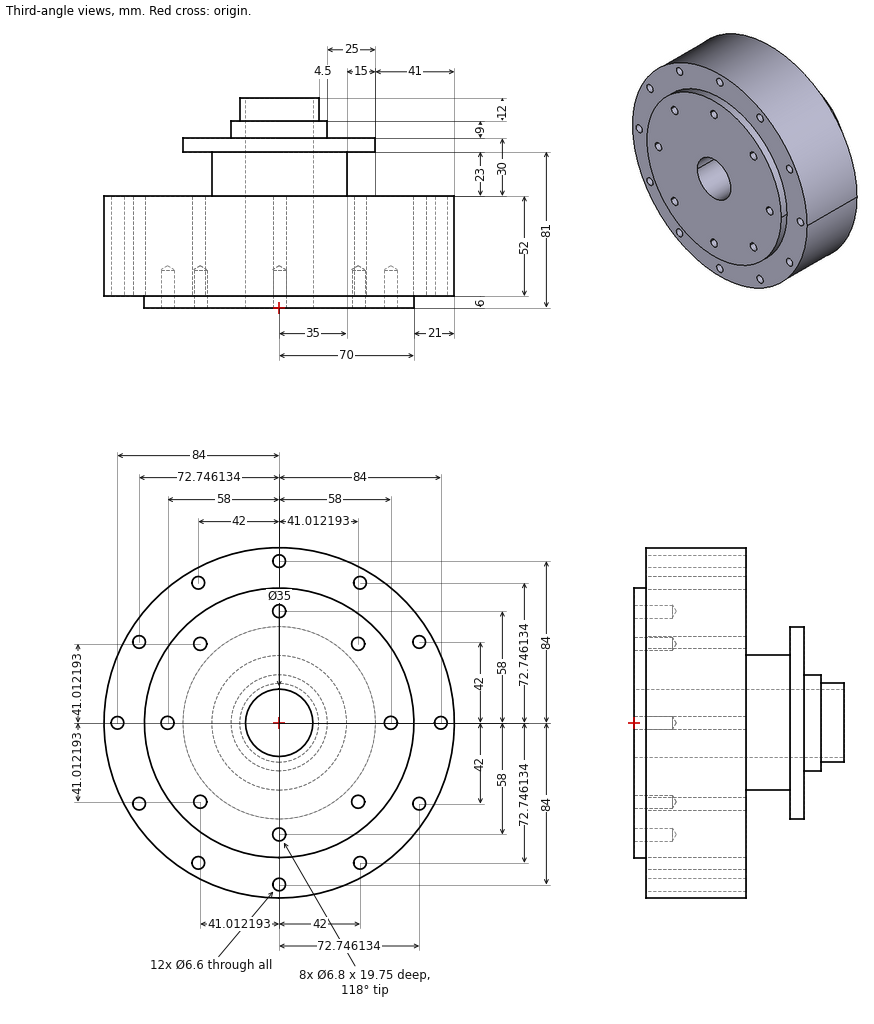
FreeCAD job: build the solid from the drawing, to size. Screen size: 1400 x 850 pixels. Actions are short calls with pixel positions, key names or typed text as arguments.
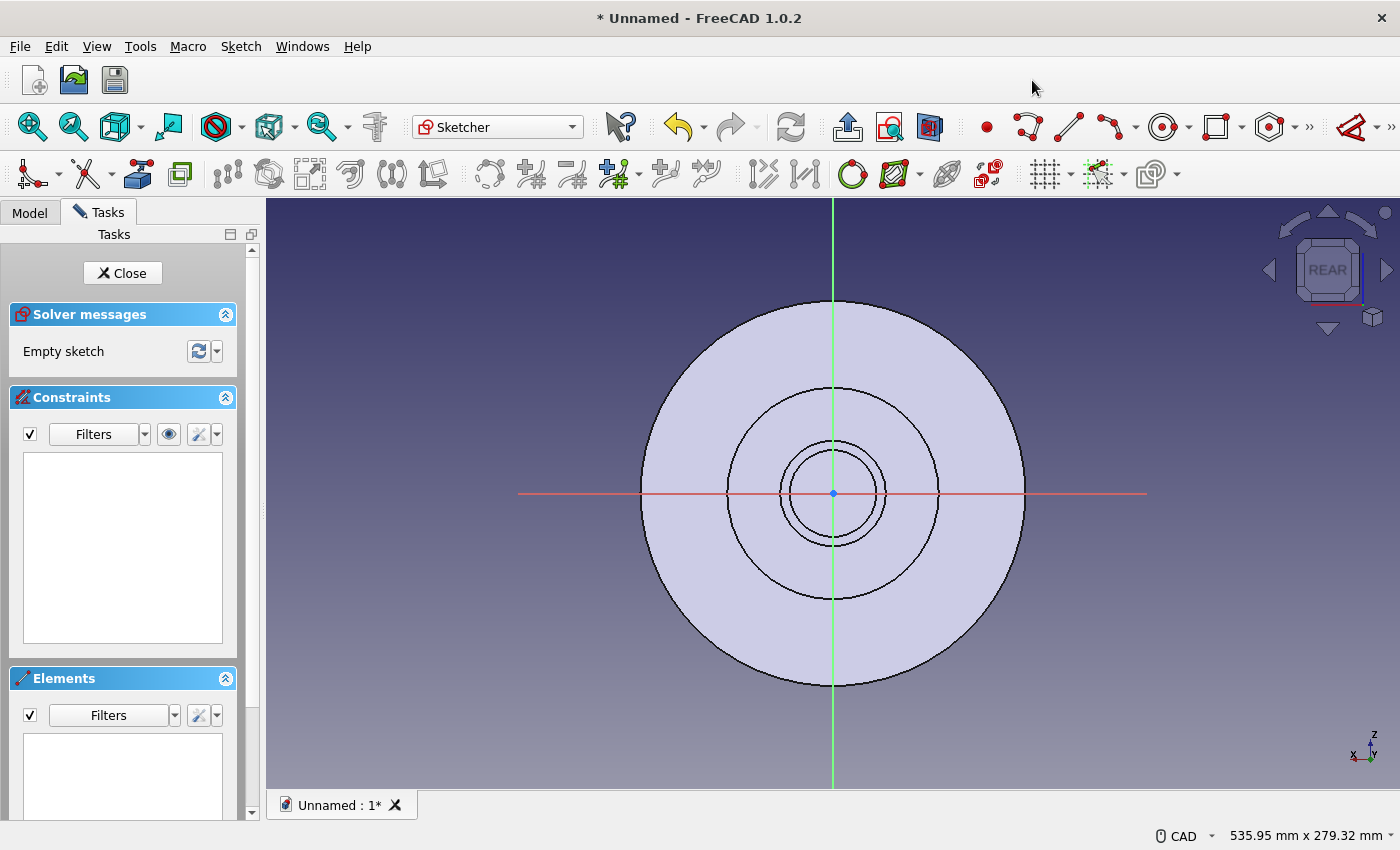
scroll(850, 493, up, 8)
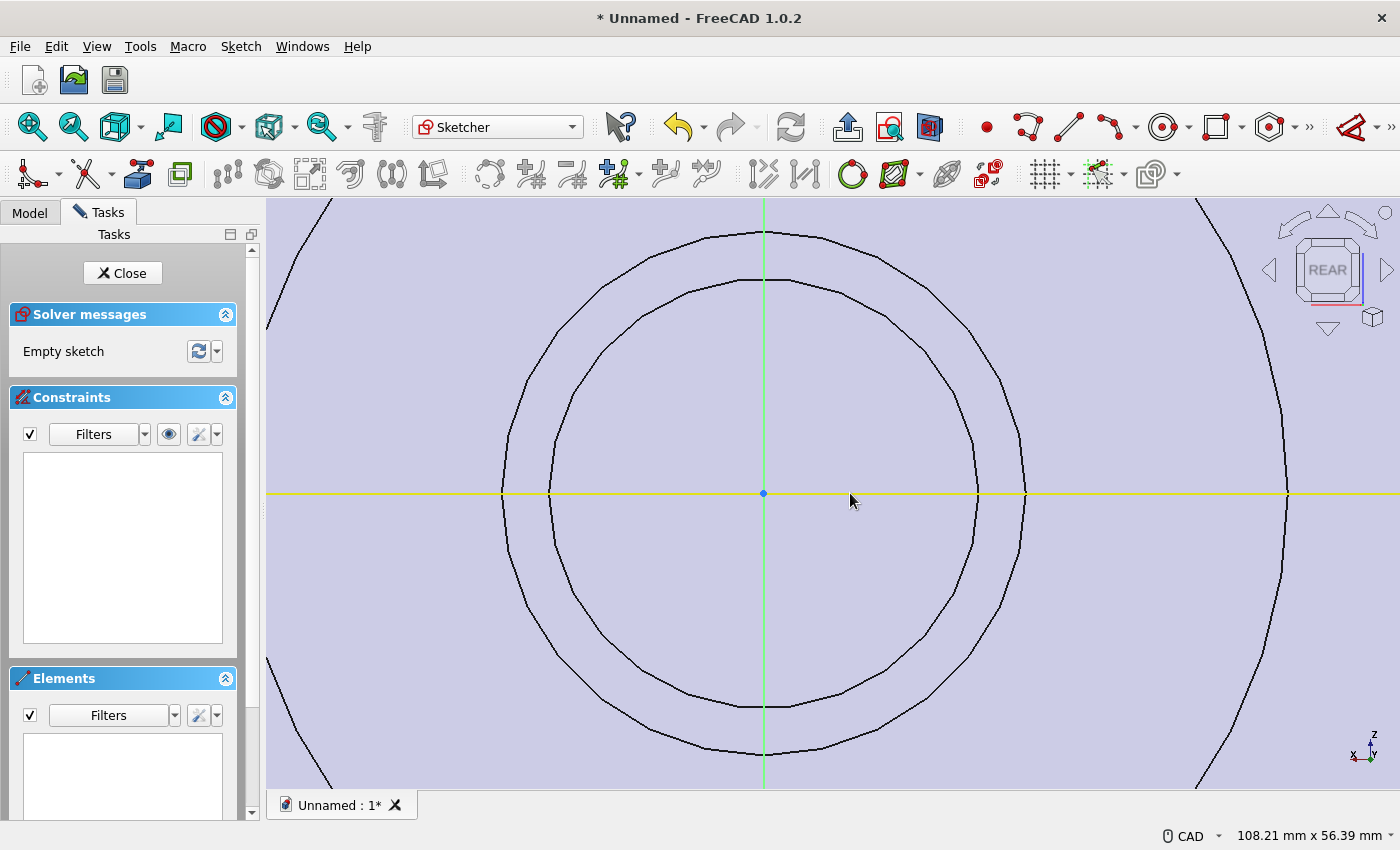
key(g)
key(c)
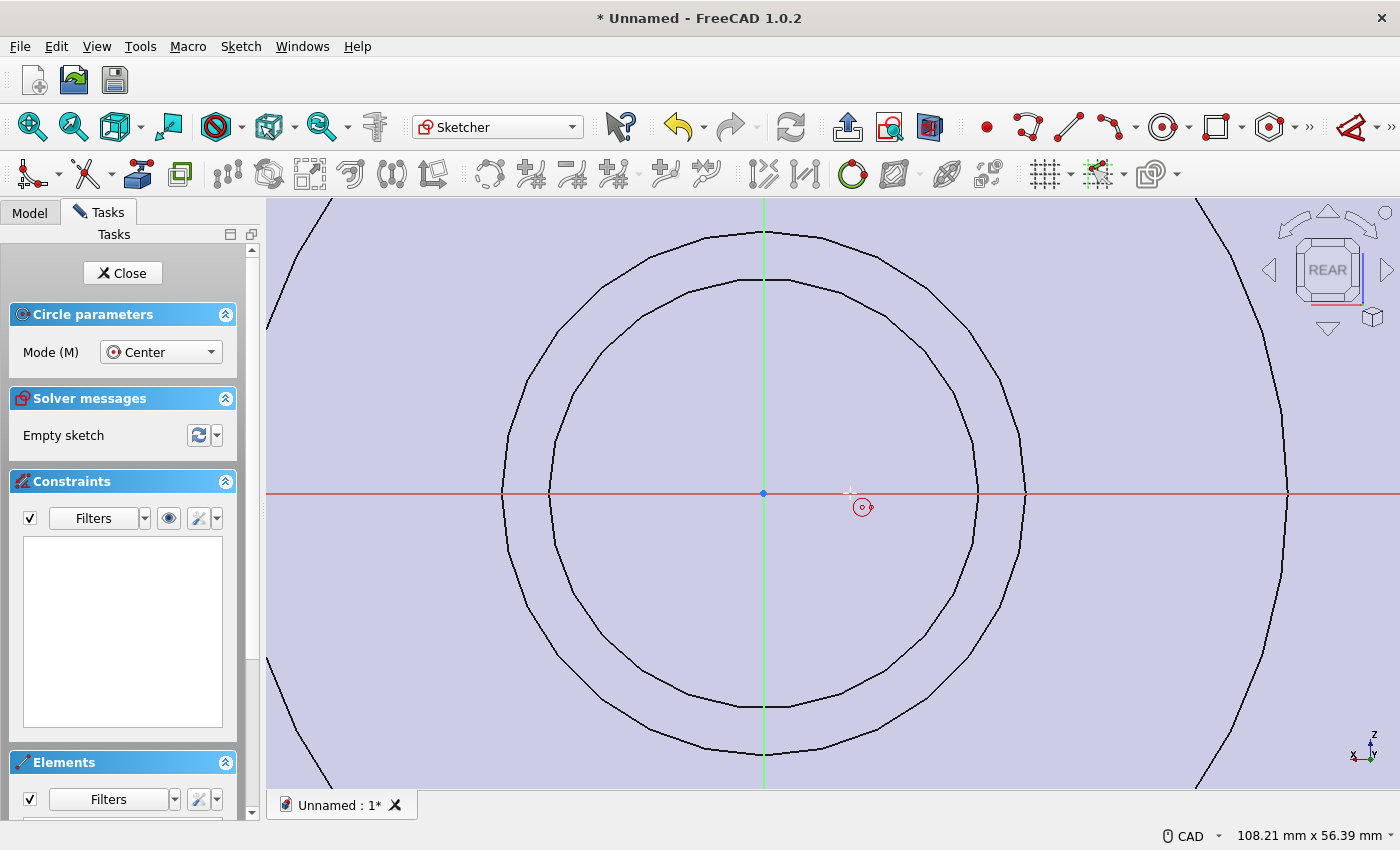
click(764, 493)
click(893, 364)
key(Escape)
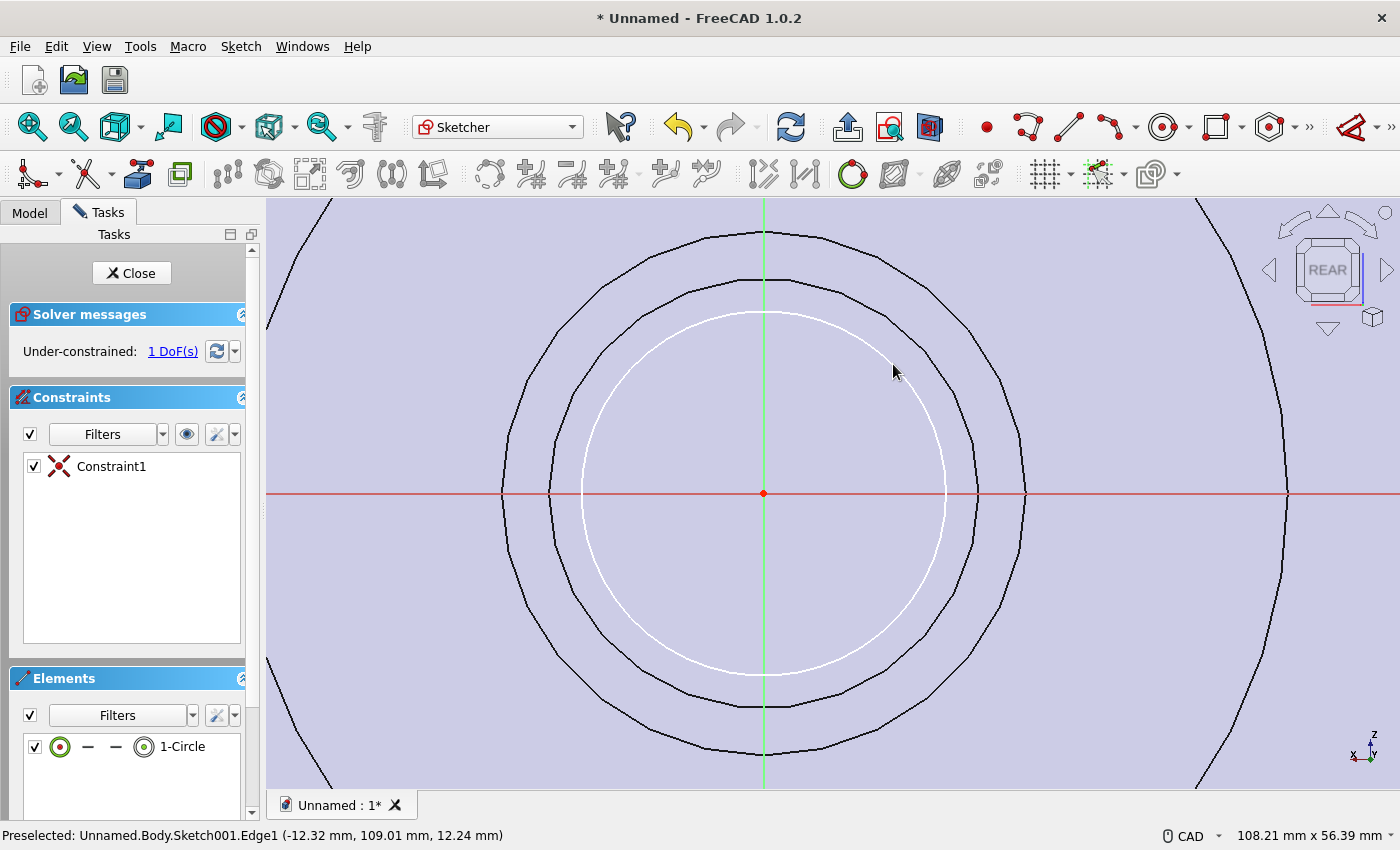
key(d)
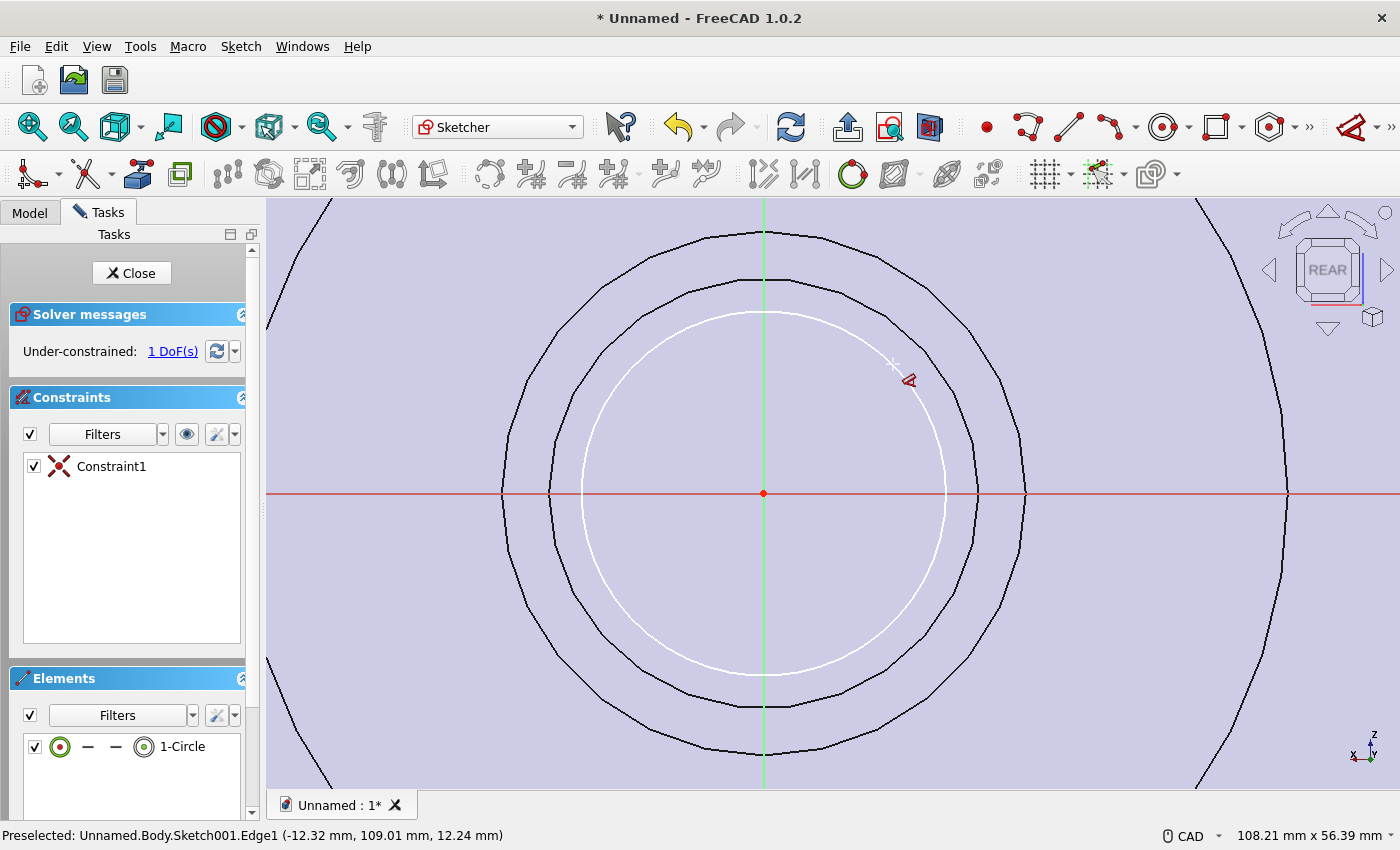
click(892, 364)
click(915, 341)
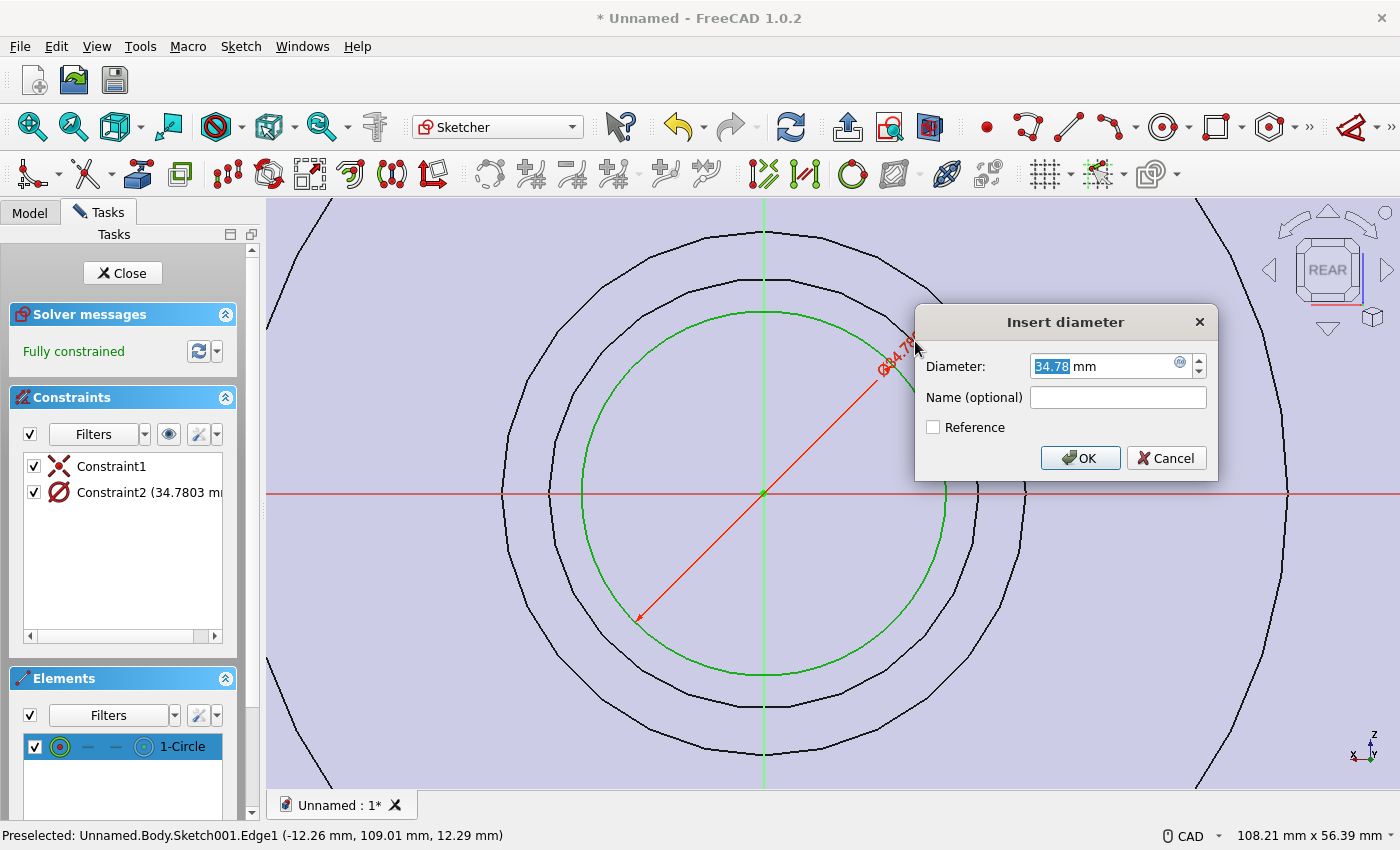
text(35)
key(Return)
key(Escape)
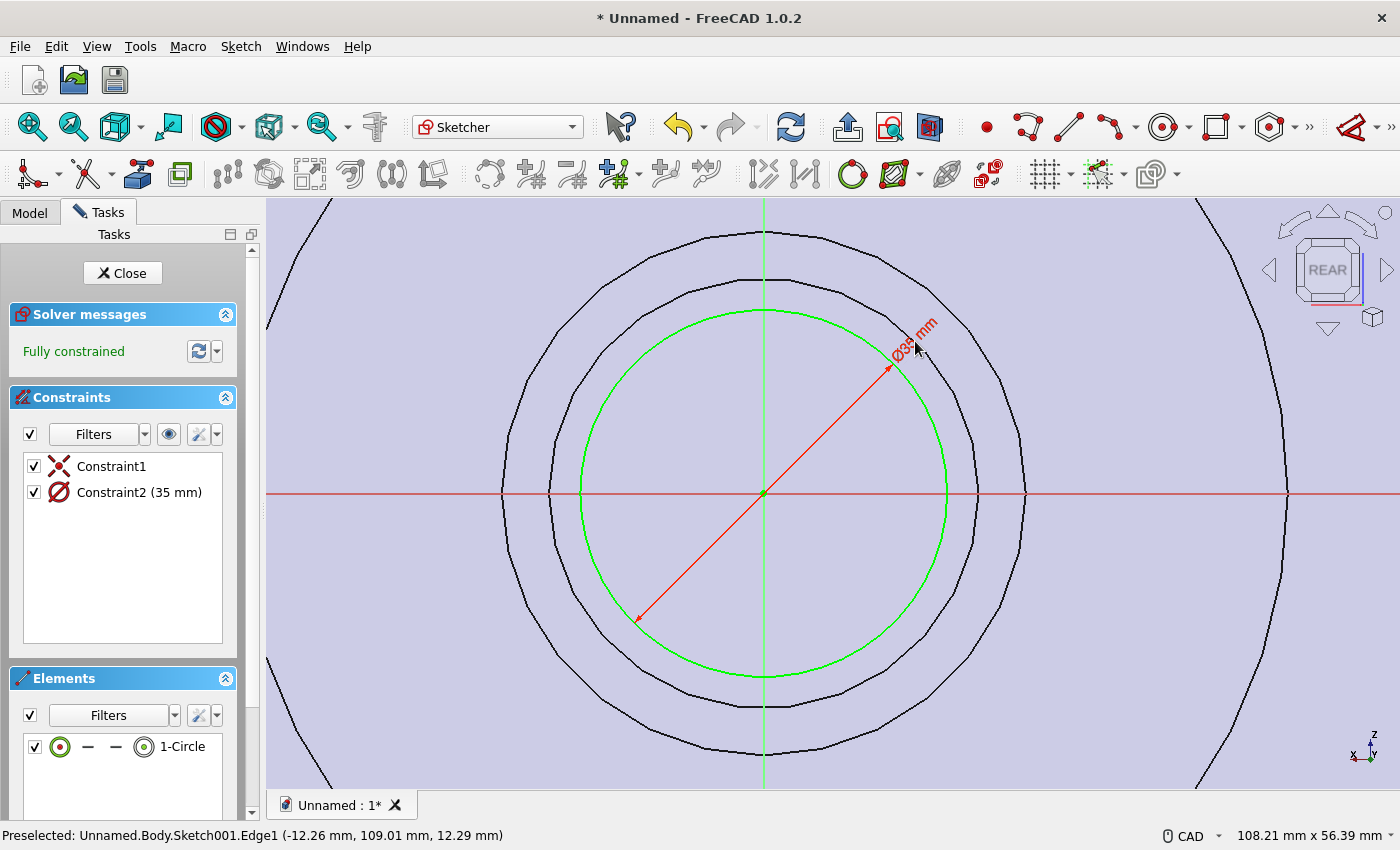
click(123, 273)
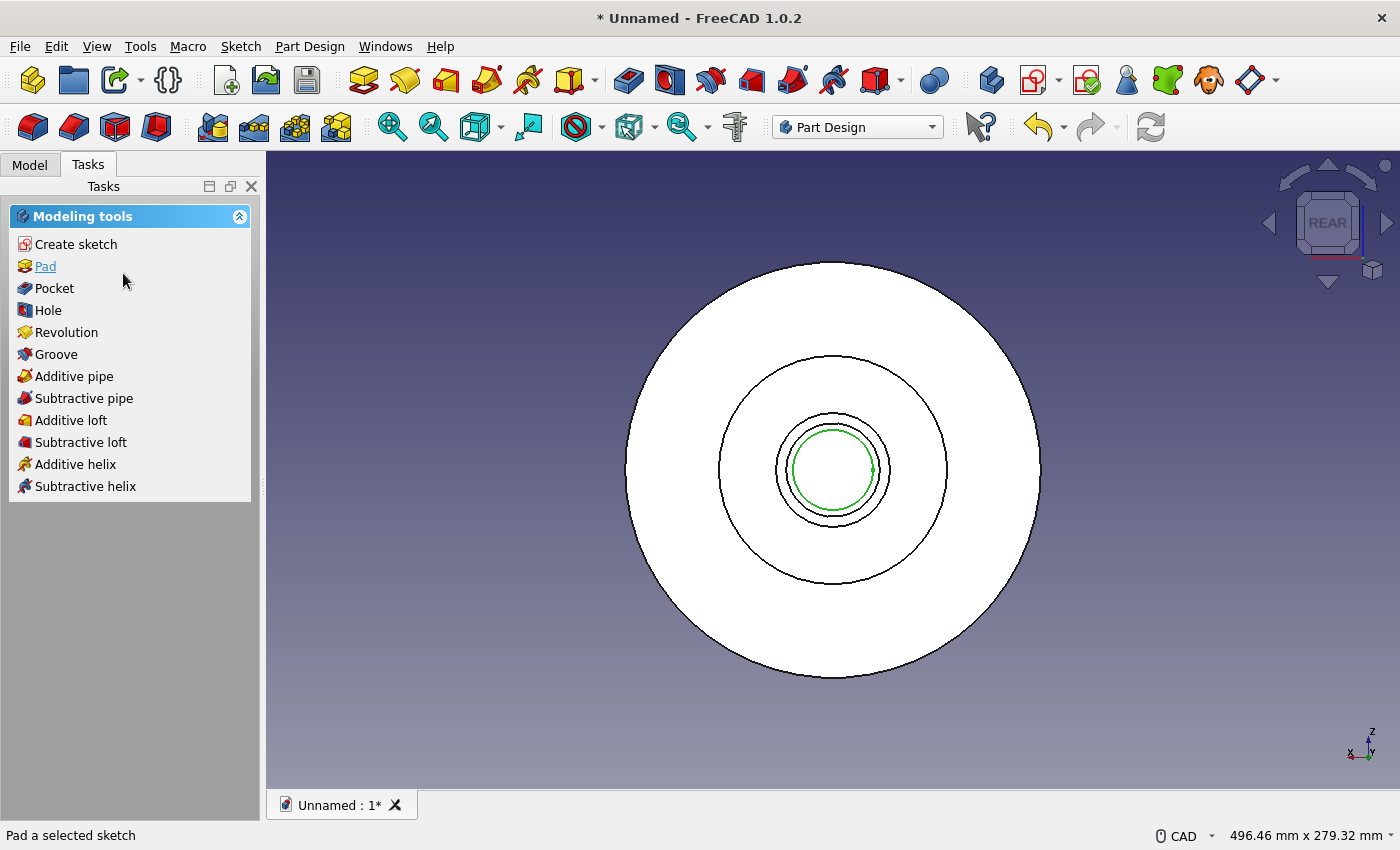
click(629, 80)